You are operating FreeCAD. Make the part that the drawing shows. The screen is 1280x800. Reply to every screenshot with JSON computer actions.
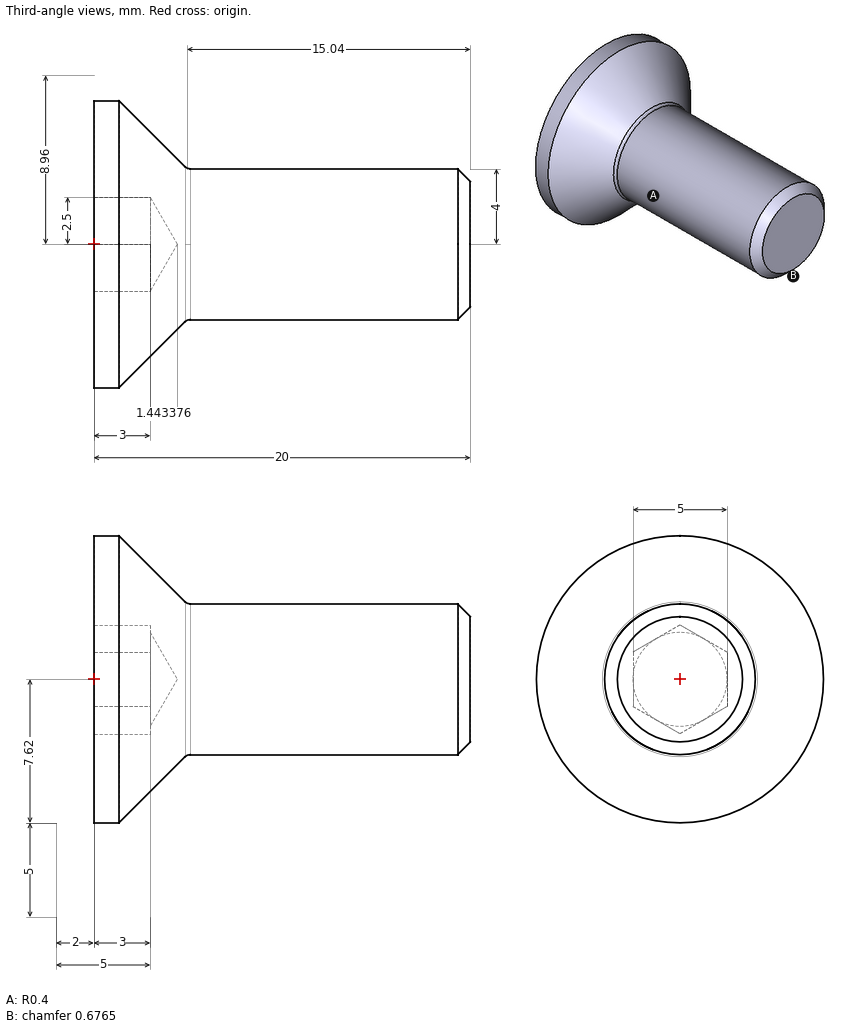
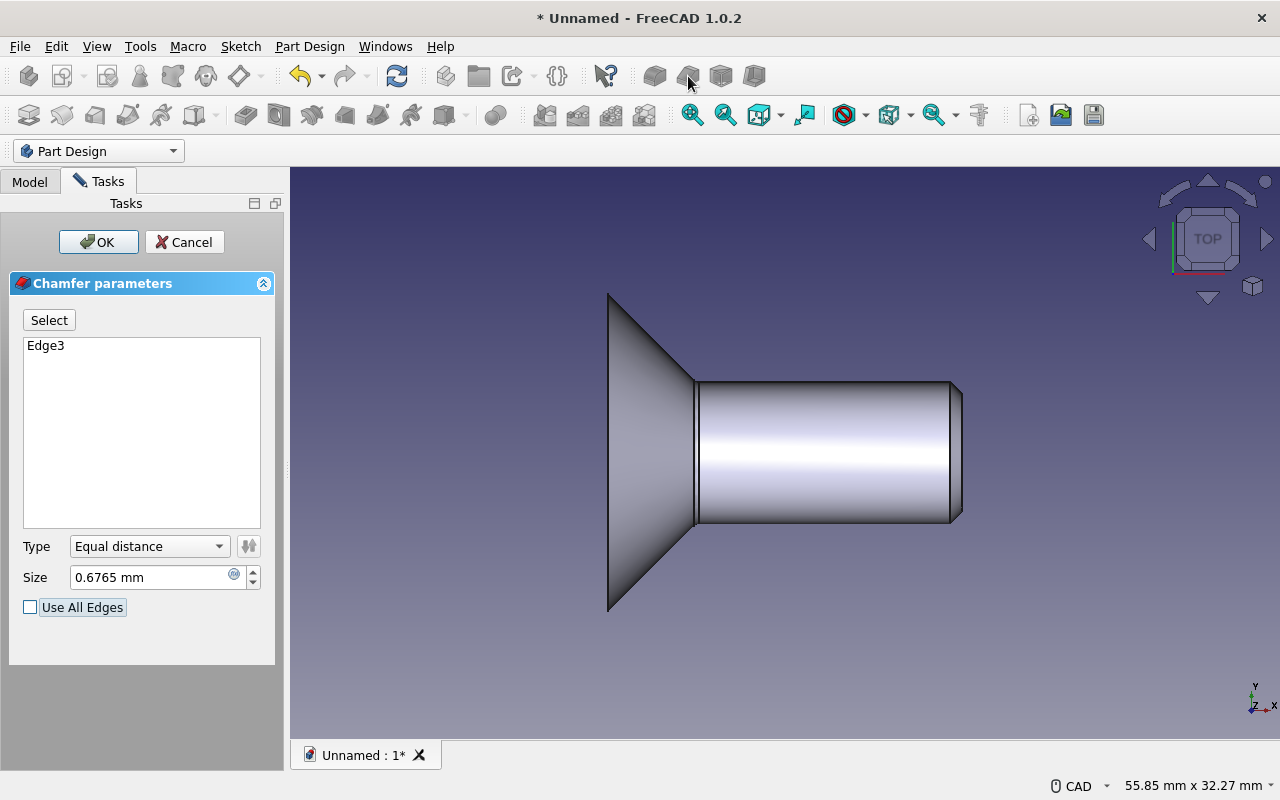
{"action": "left_click", "coordinate": [99, 242]}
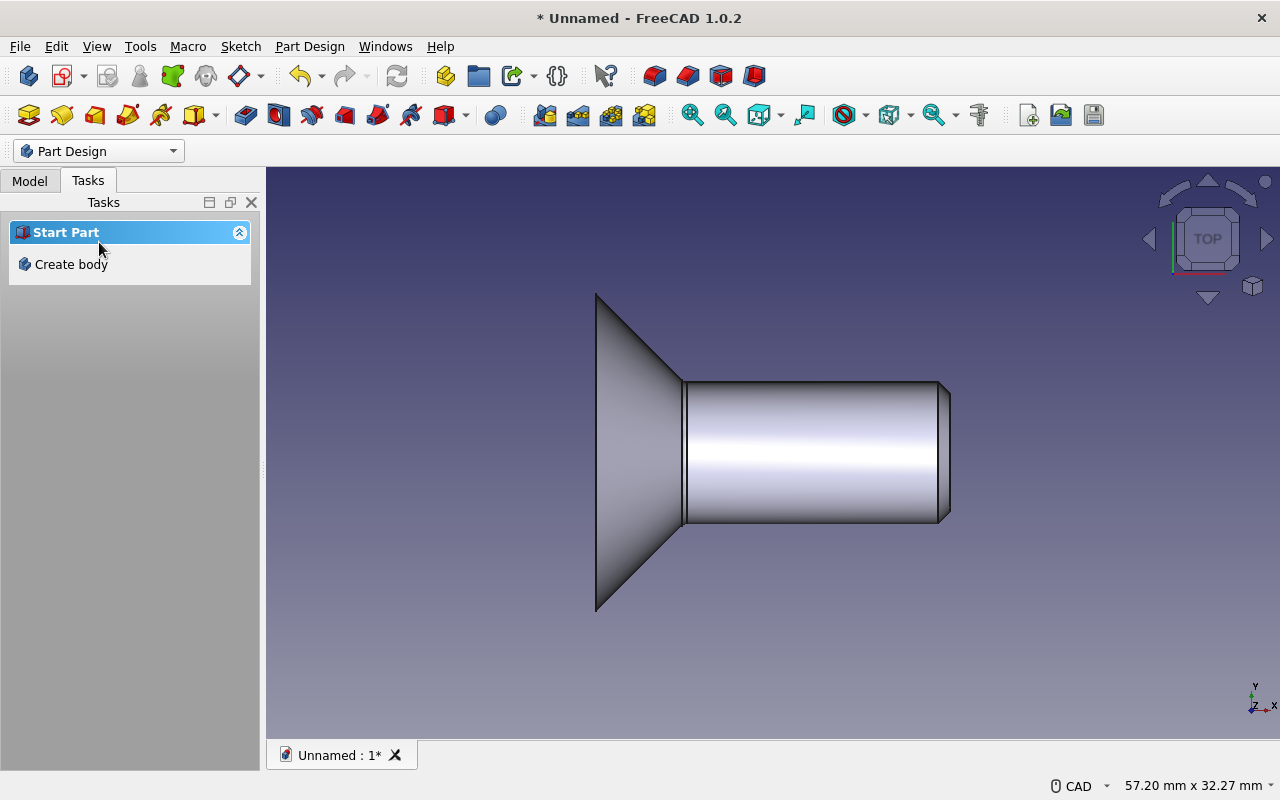
{"action": "left_click", "coordinate": [62, 76]}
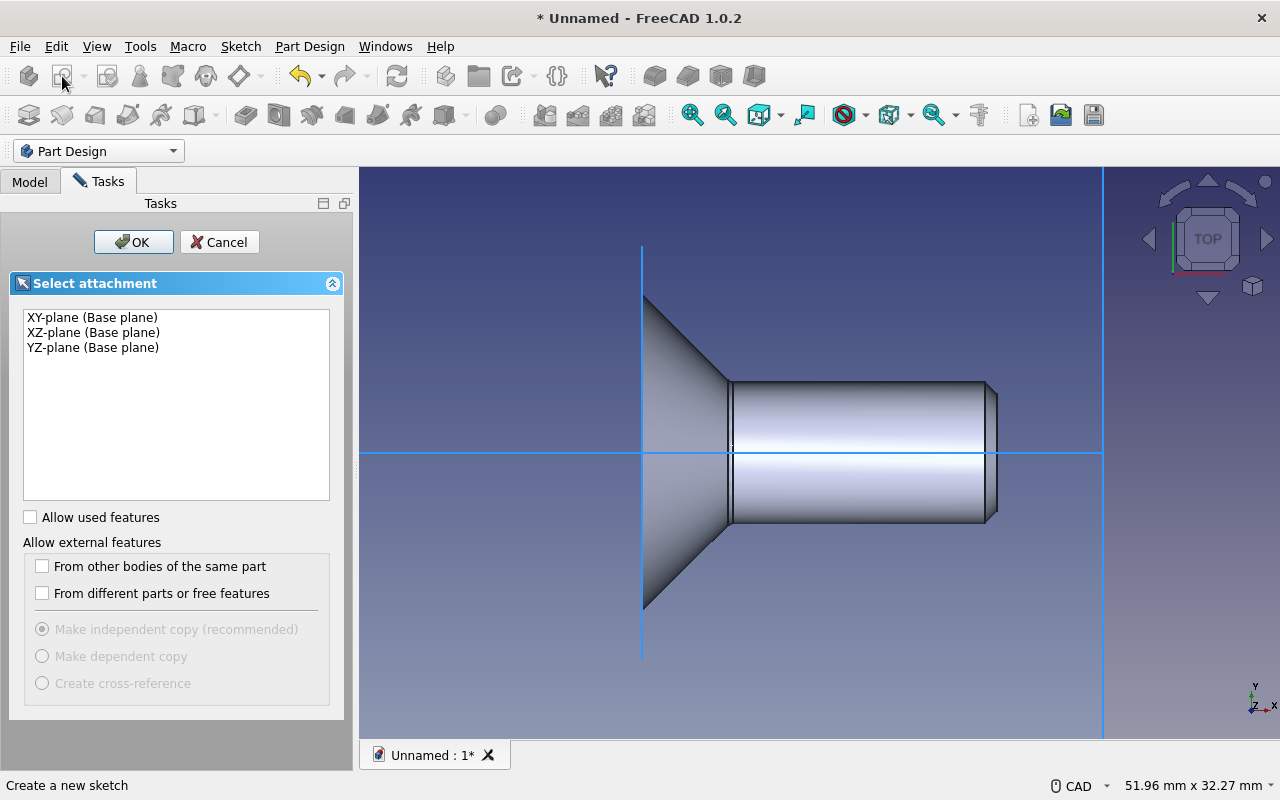
{"action": "left_click", "coordinate": [84, 332]}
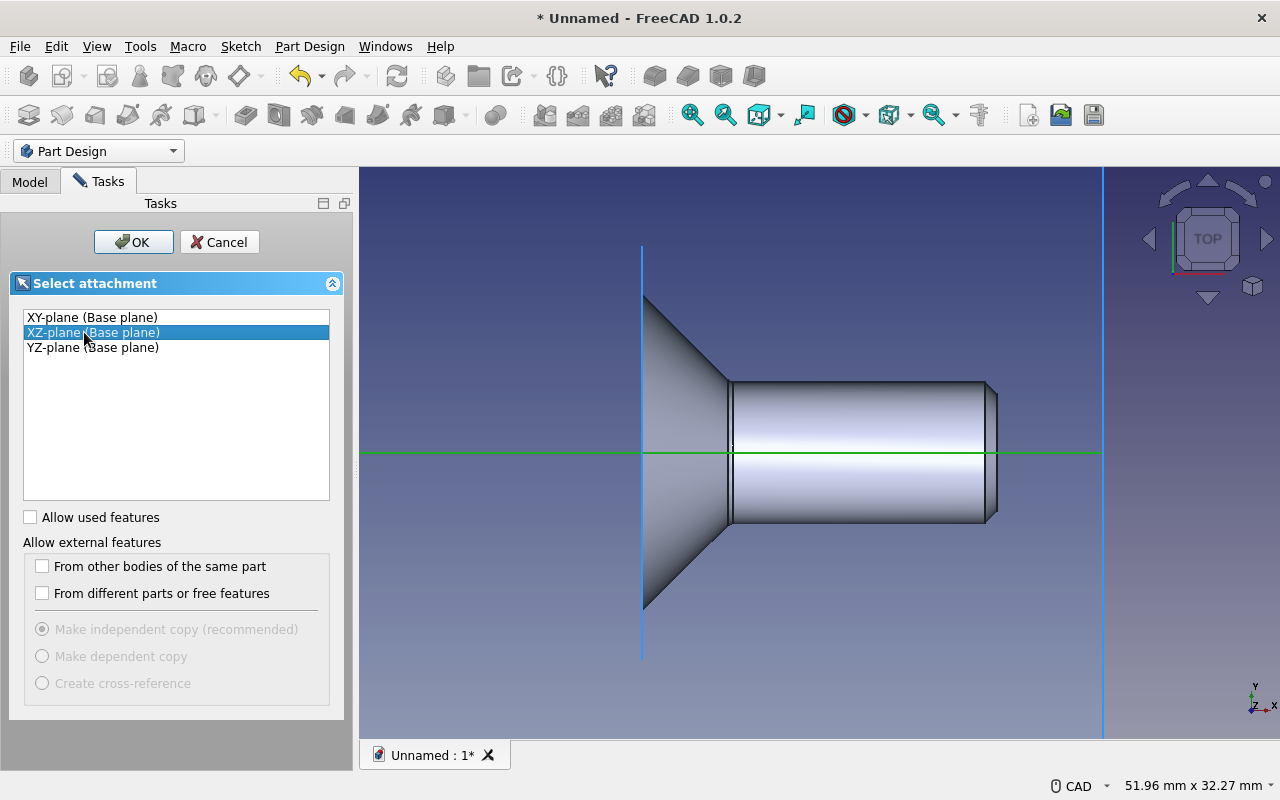
{"action": "left_click", "coordinate": [134, 242]}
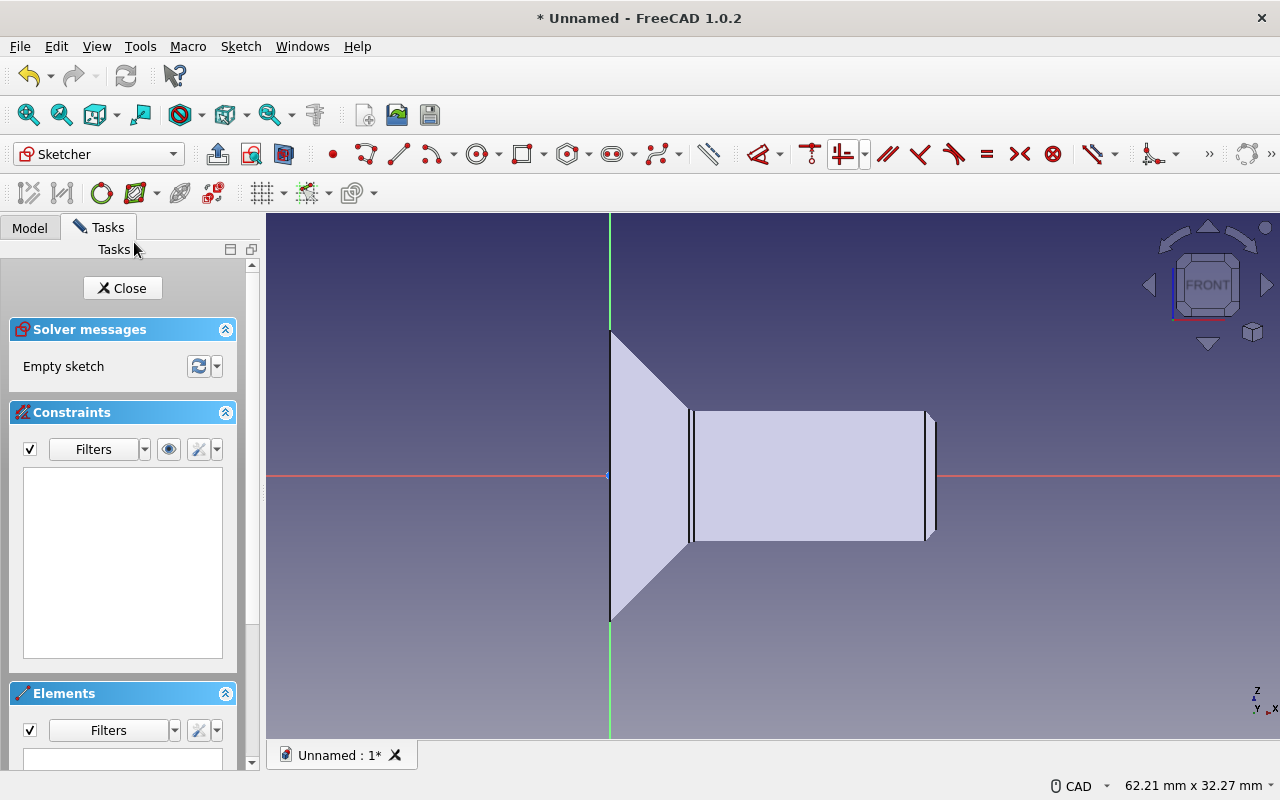
{"action": "left_click", "coordinate": [284, 154]}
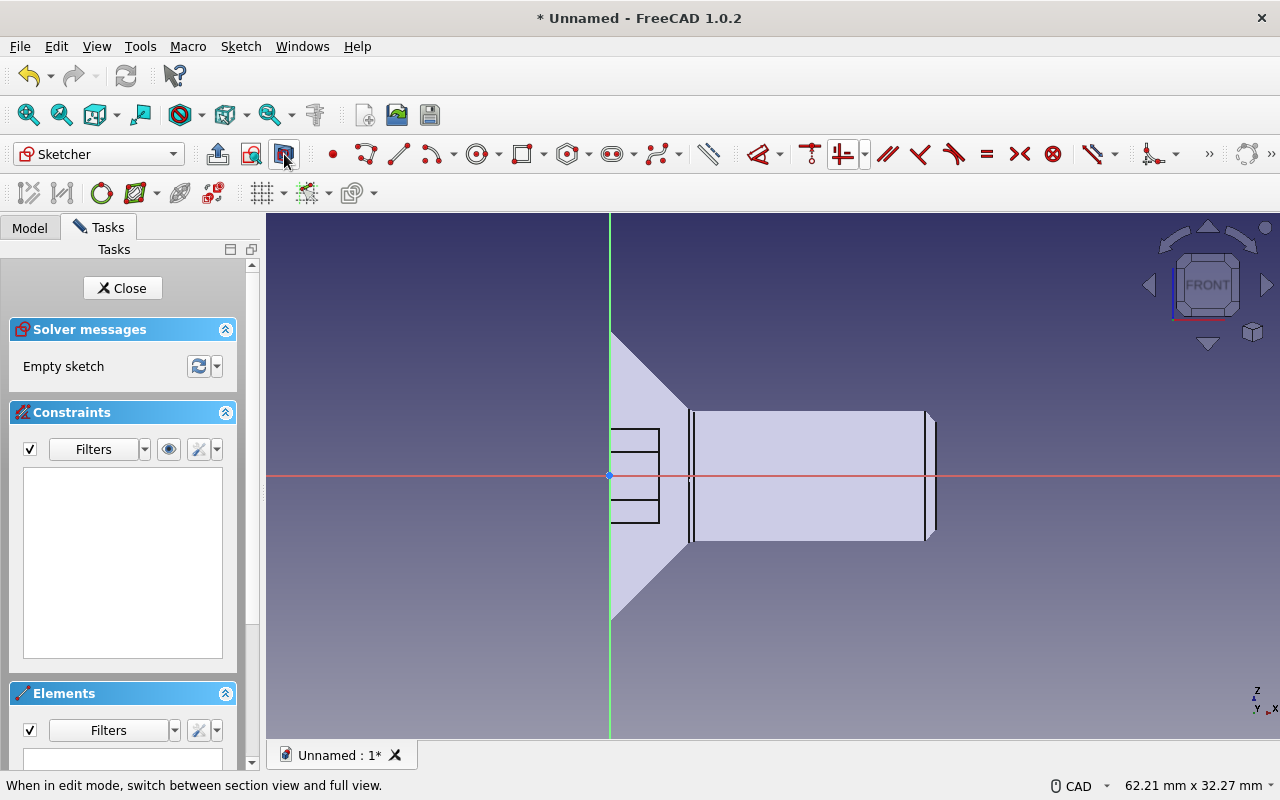
{"action": "scroll", "coordinate": [590, 695], "scroll_direction": "up", "scroll_amount": 7}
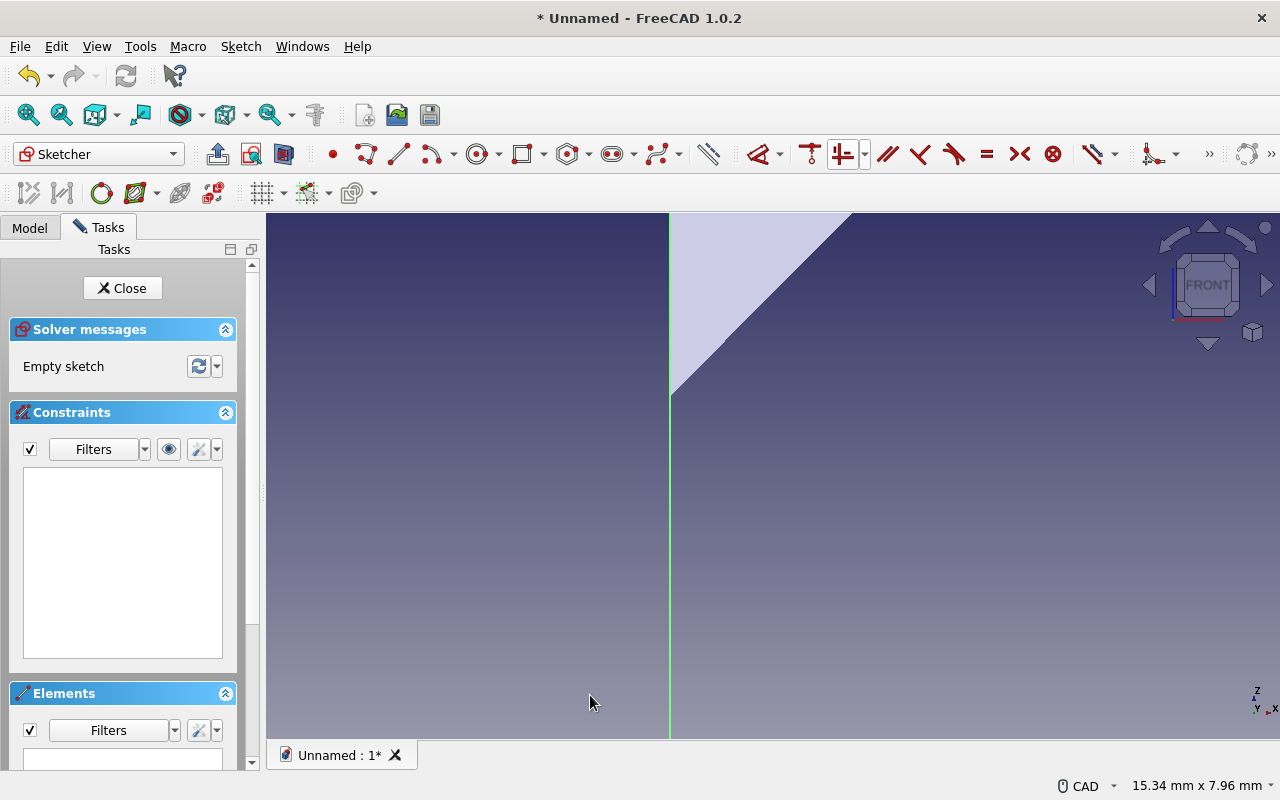
{"action": "left_click", "coordinate": [522, 154]}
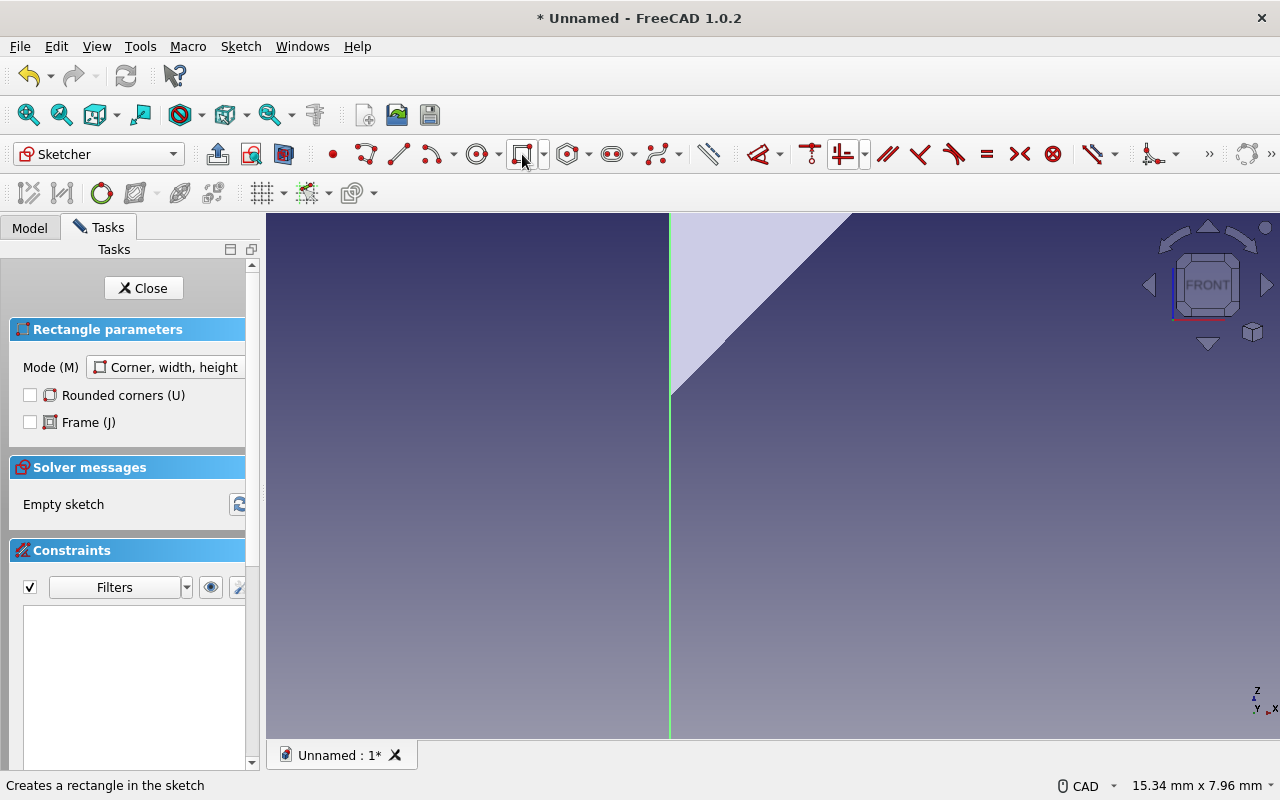
{"action": "left_click", "coordinate": [538, 308]}
{"action": "left_click", "coordinate": [868, 638]}
{"action": "key", "text": "Escape"}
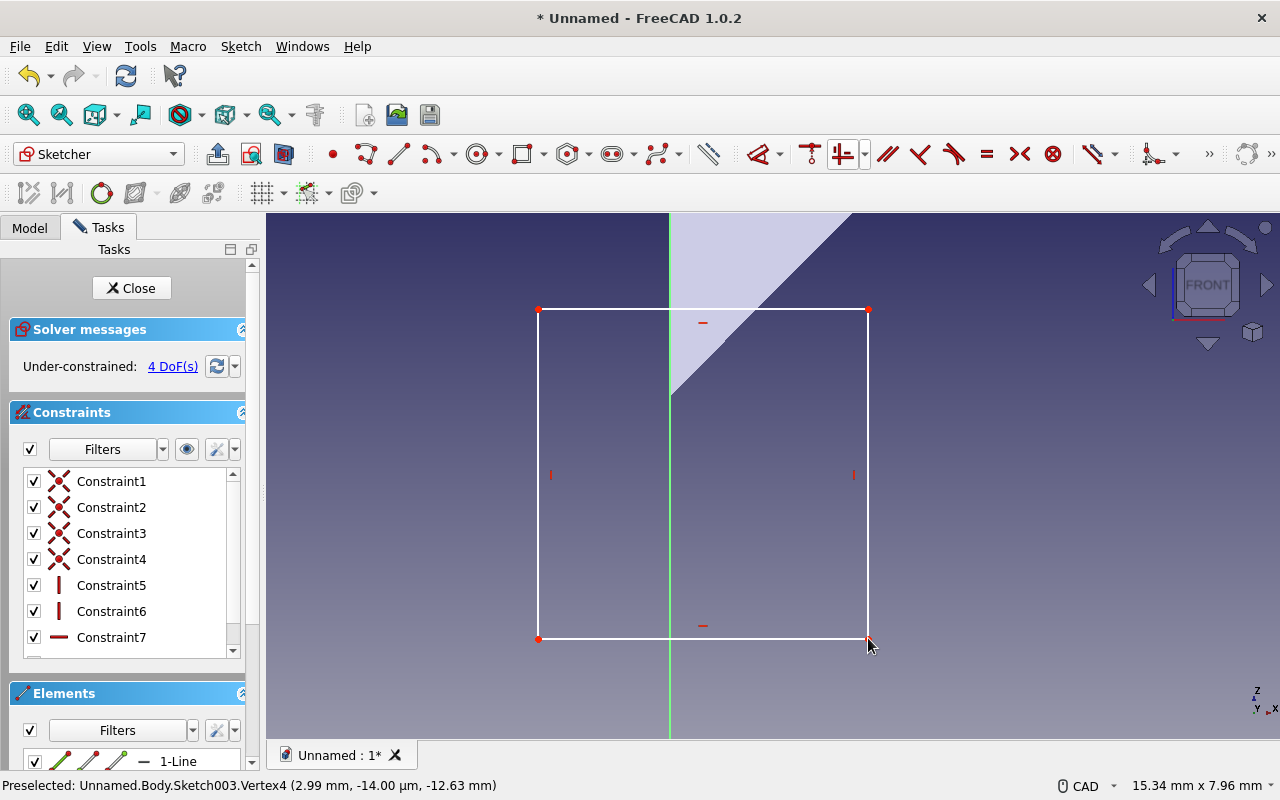
{"action": "left_click", "coordinate": [758, 154]}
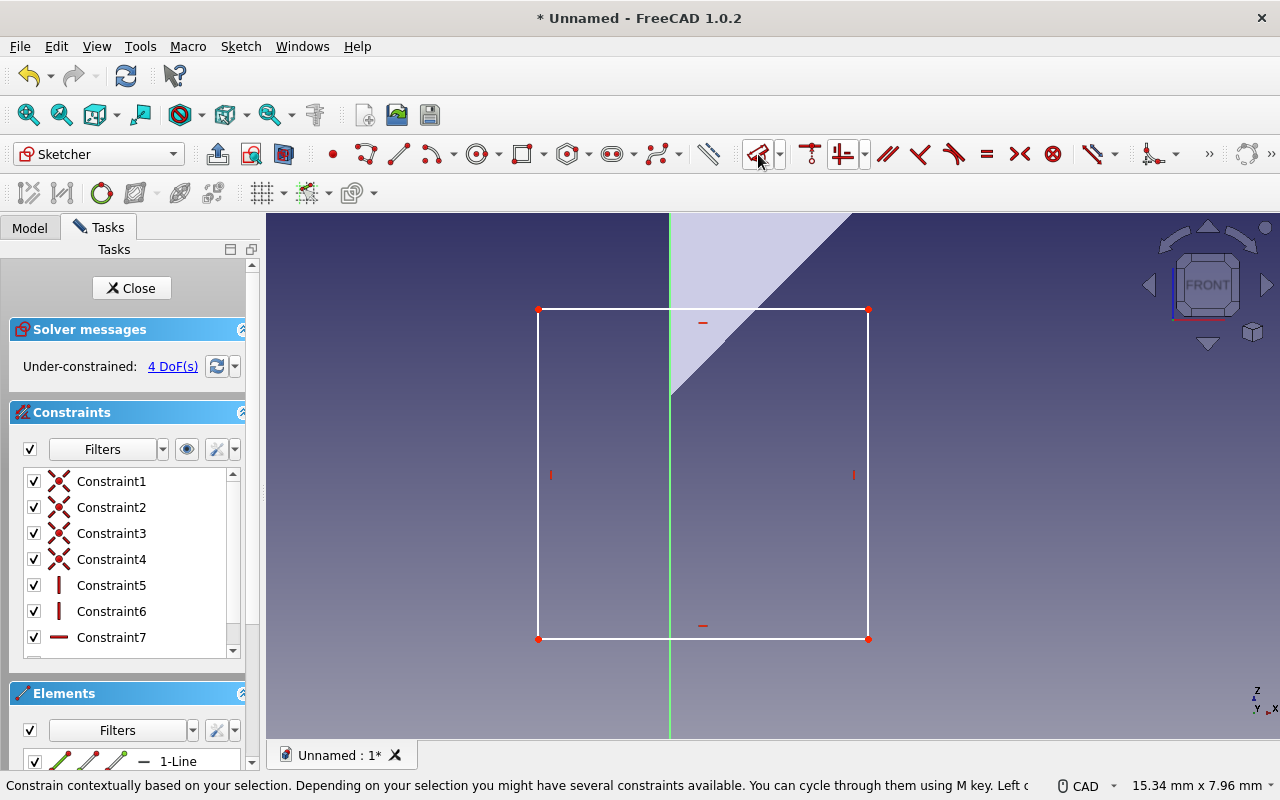
{"action": "left_click", "coordinate": [538, 408]}
{"action": "left_click", "coordinate": [504, 474]}